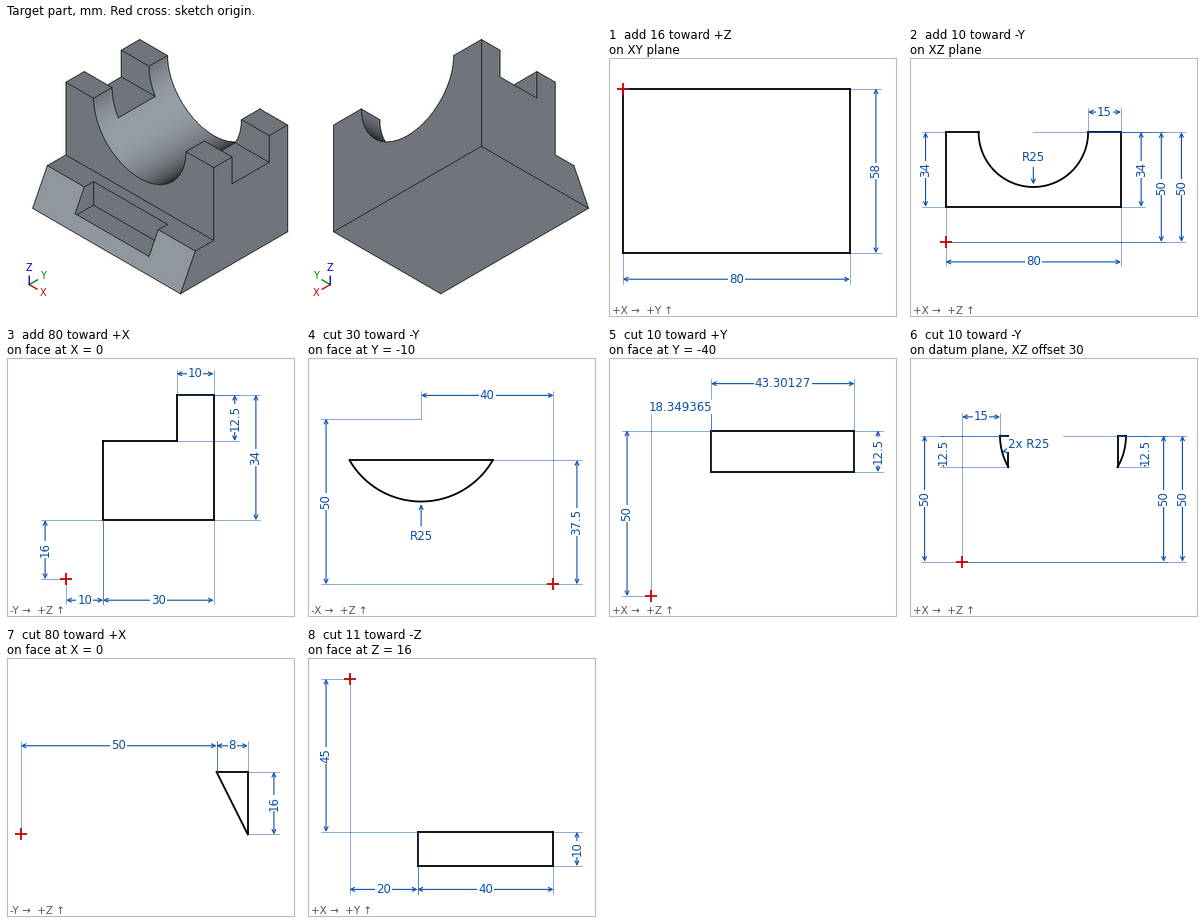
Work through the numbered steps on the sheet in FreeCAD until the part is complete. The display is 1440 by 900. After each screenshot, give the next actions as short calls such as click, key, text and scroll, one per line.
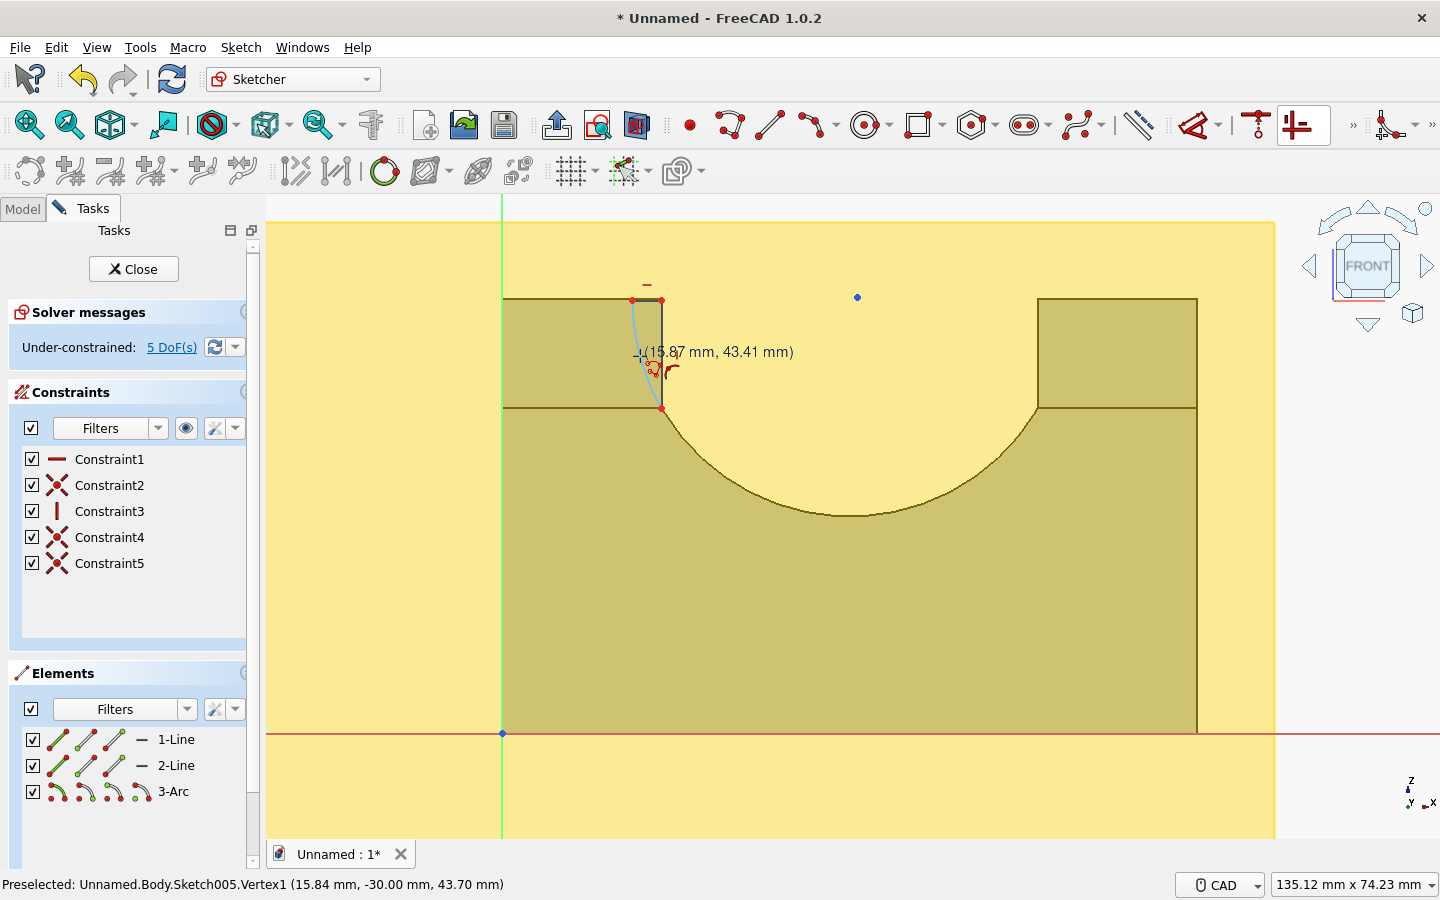
click(1038, 408)
click(1038, 299)
click(1067, 299)
right_click(1067, 299)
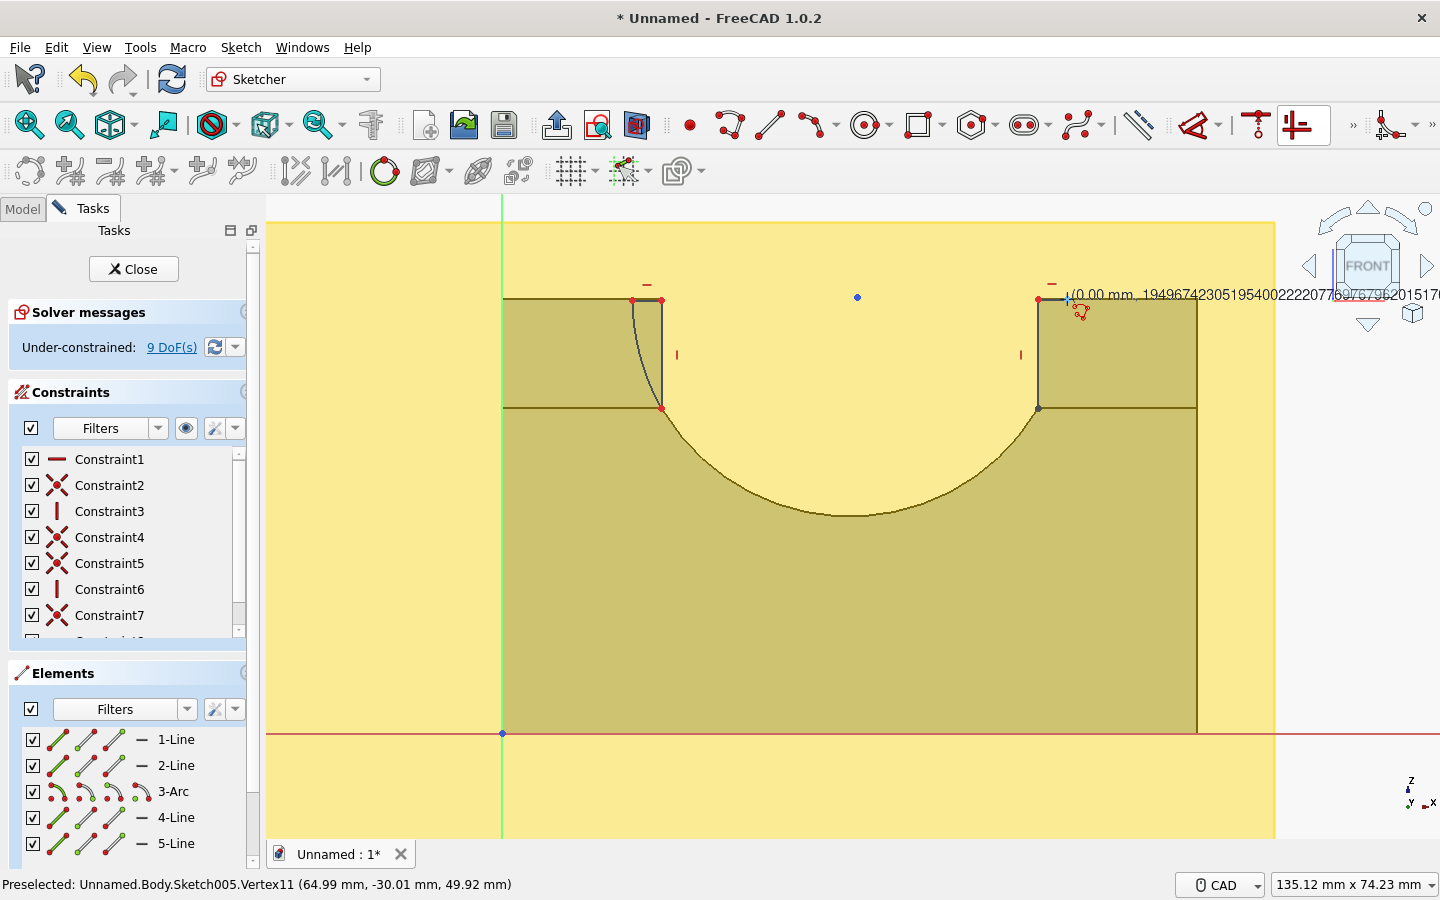
click(812, 126)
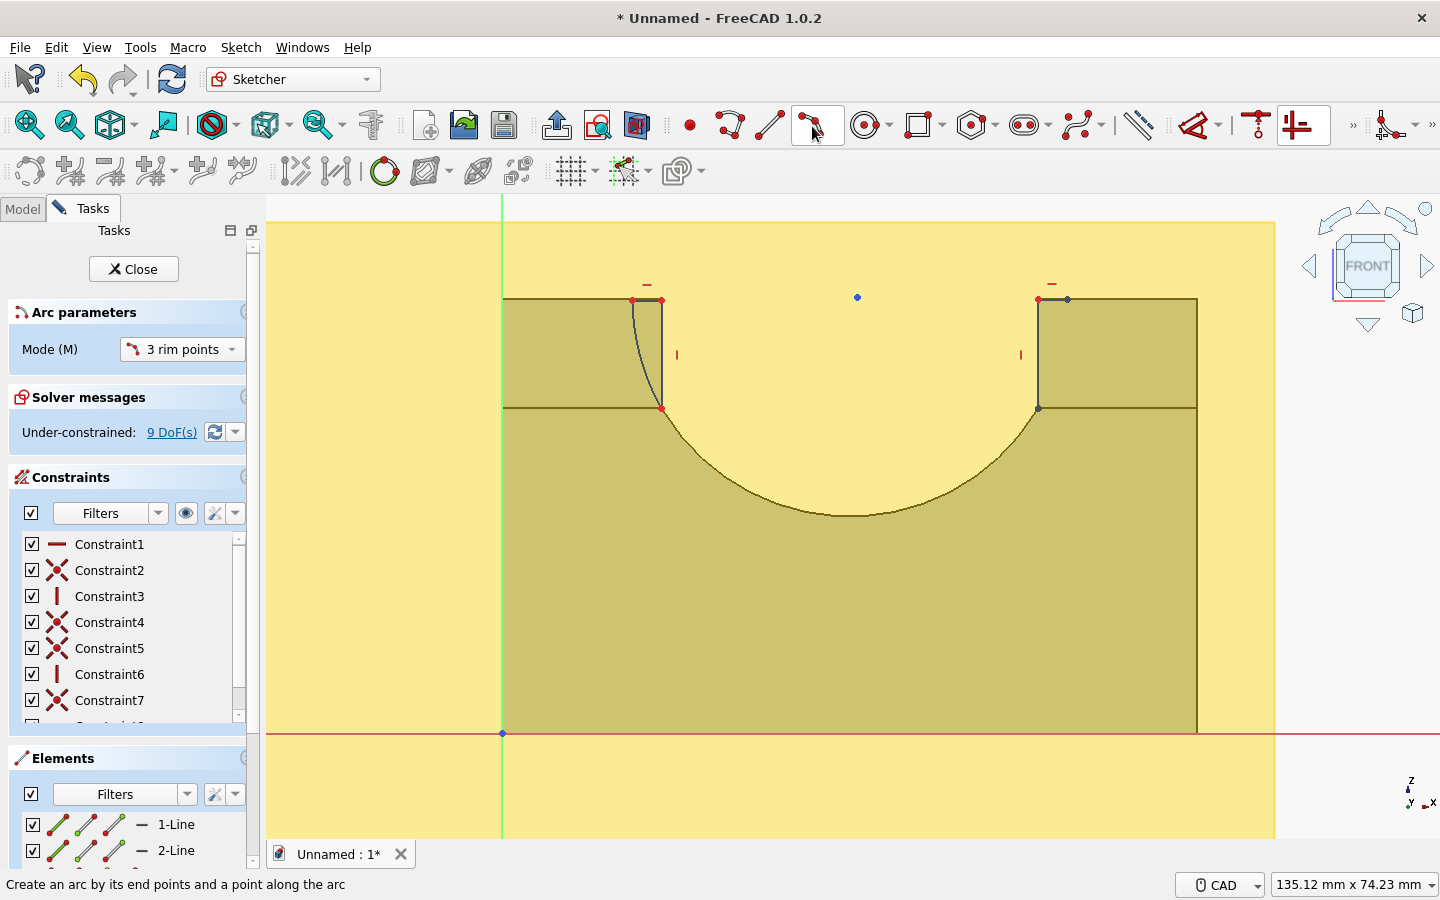
click(1067, 300)
click(1038, 409)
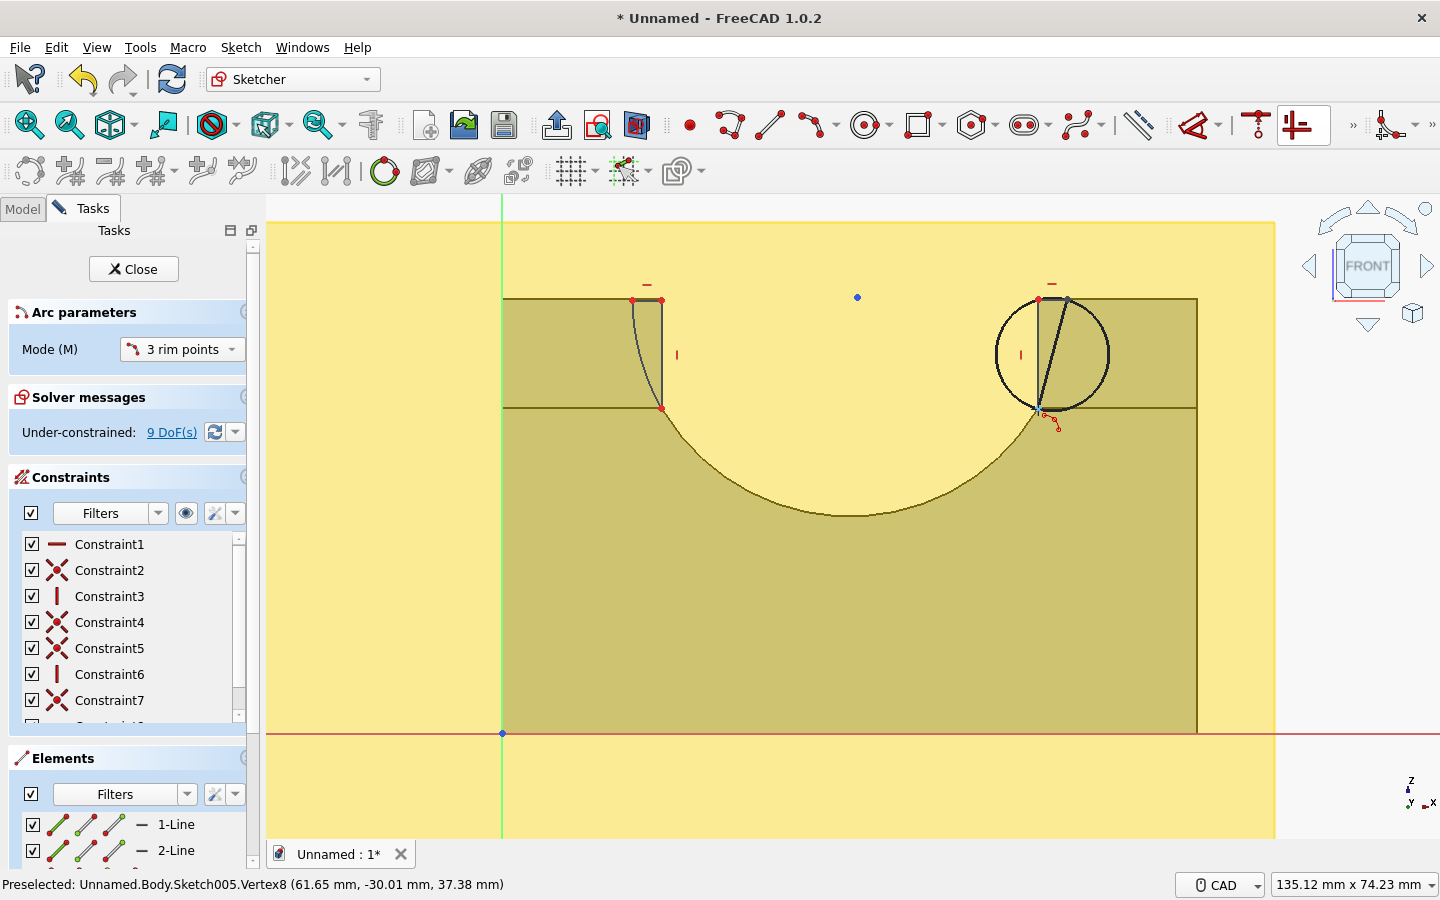
scroll(1060, 356, up, 4)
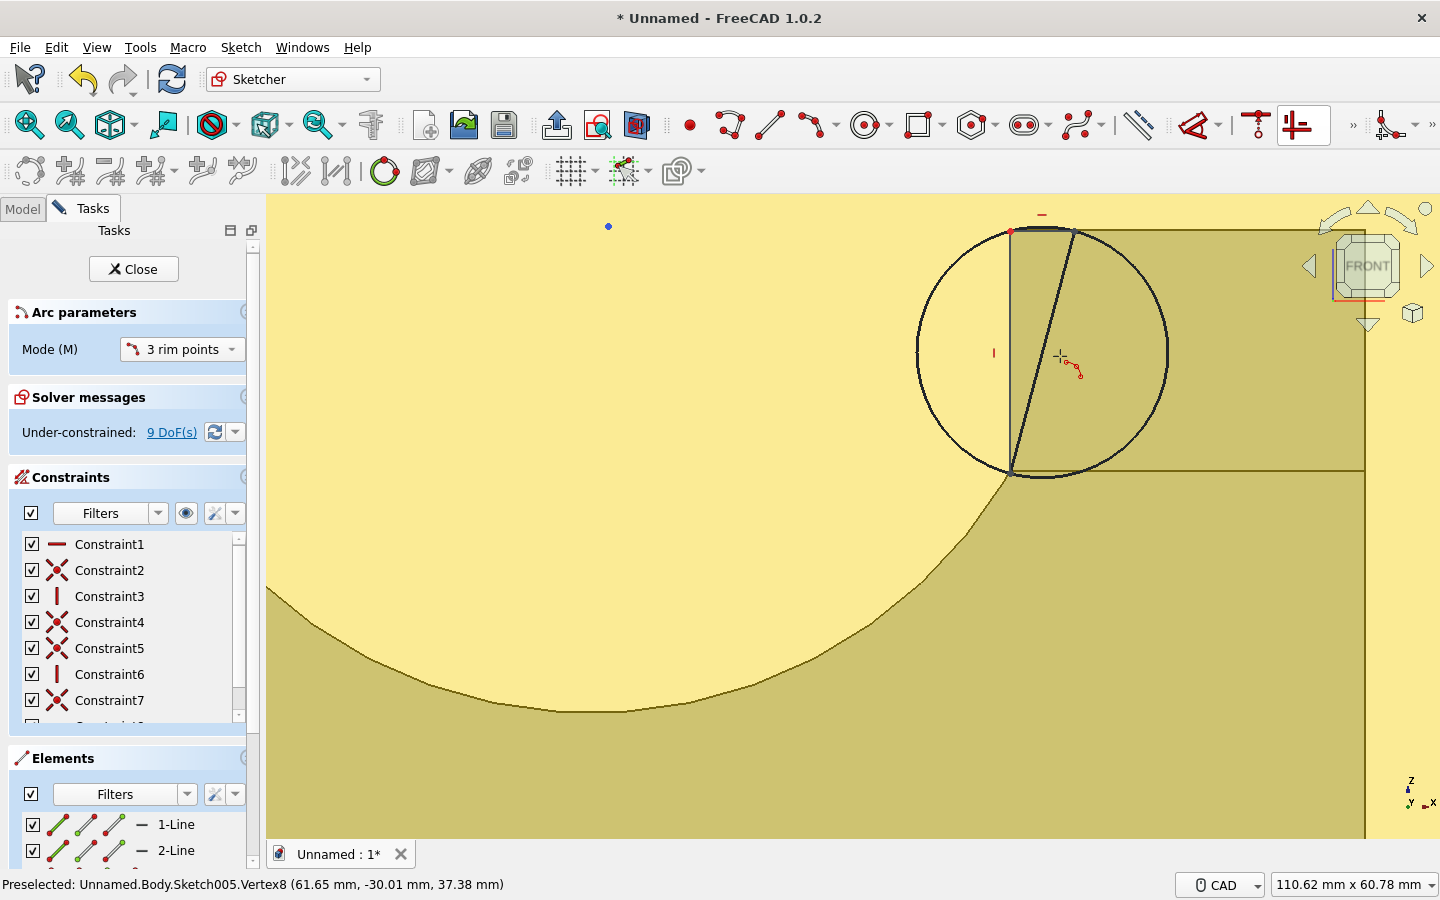
click(1058, 355)
key(Escape)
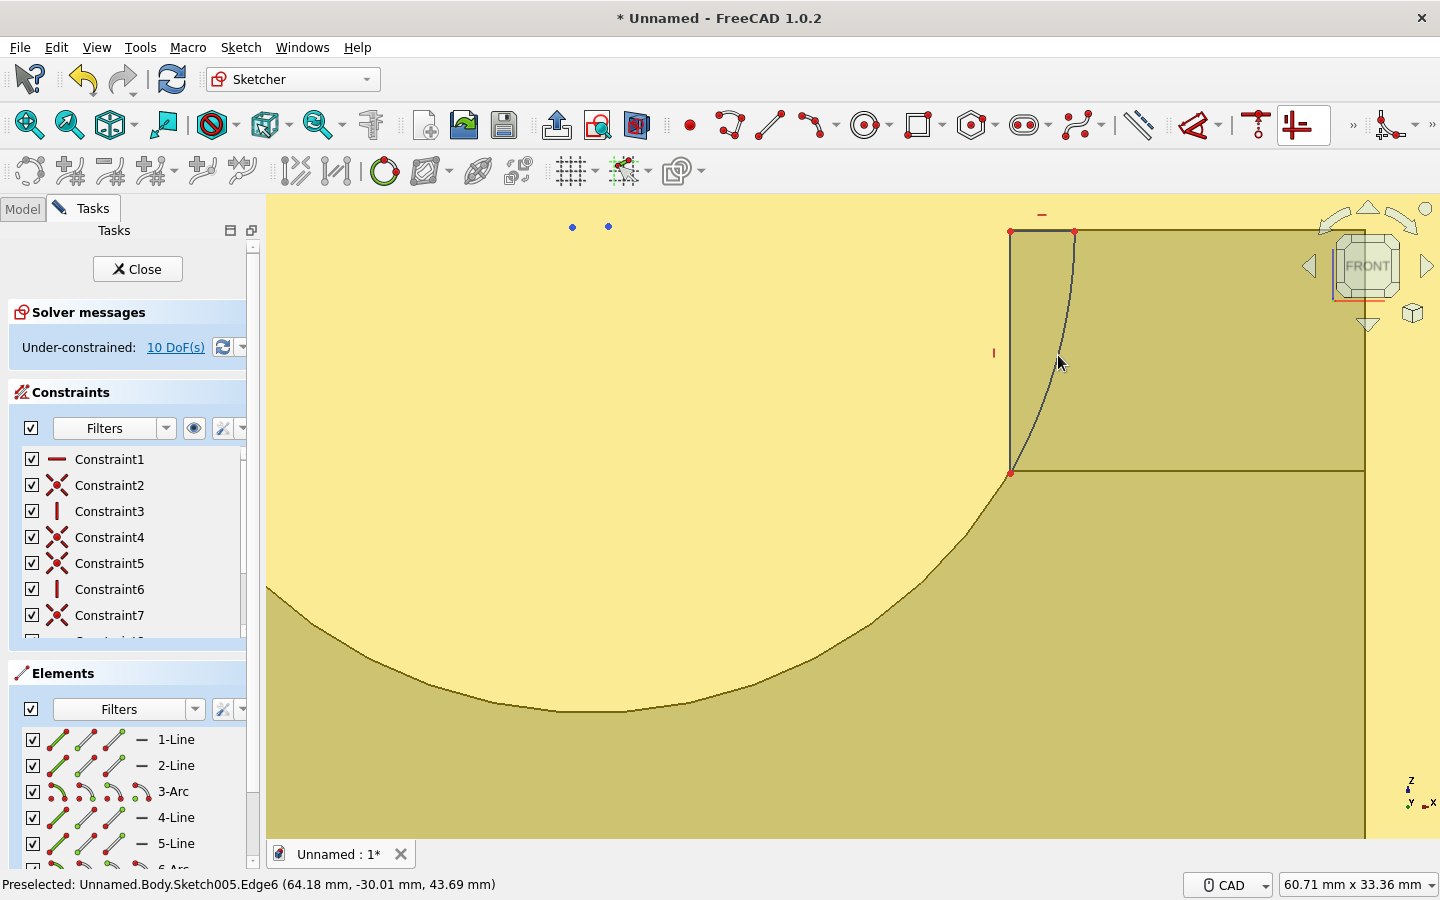
scroll(1060, 356, down, 4)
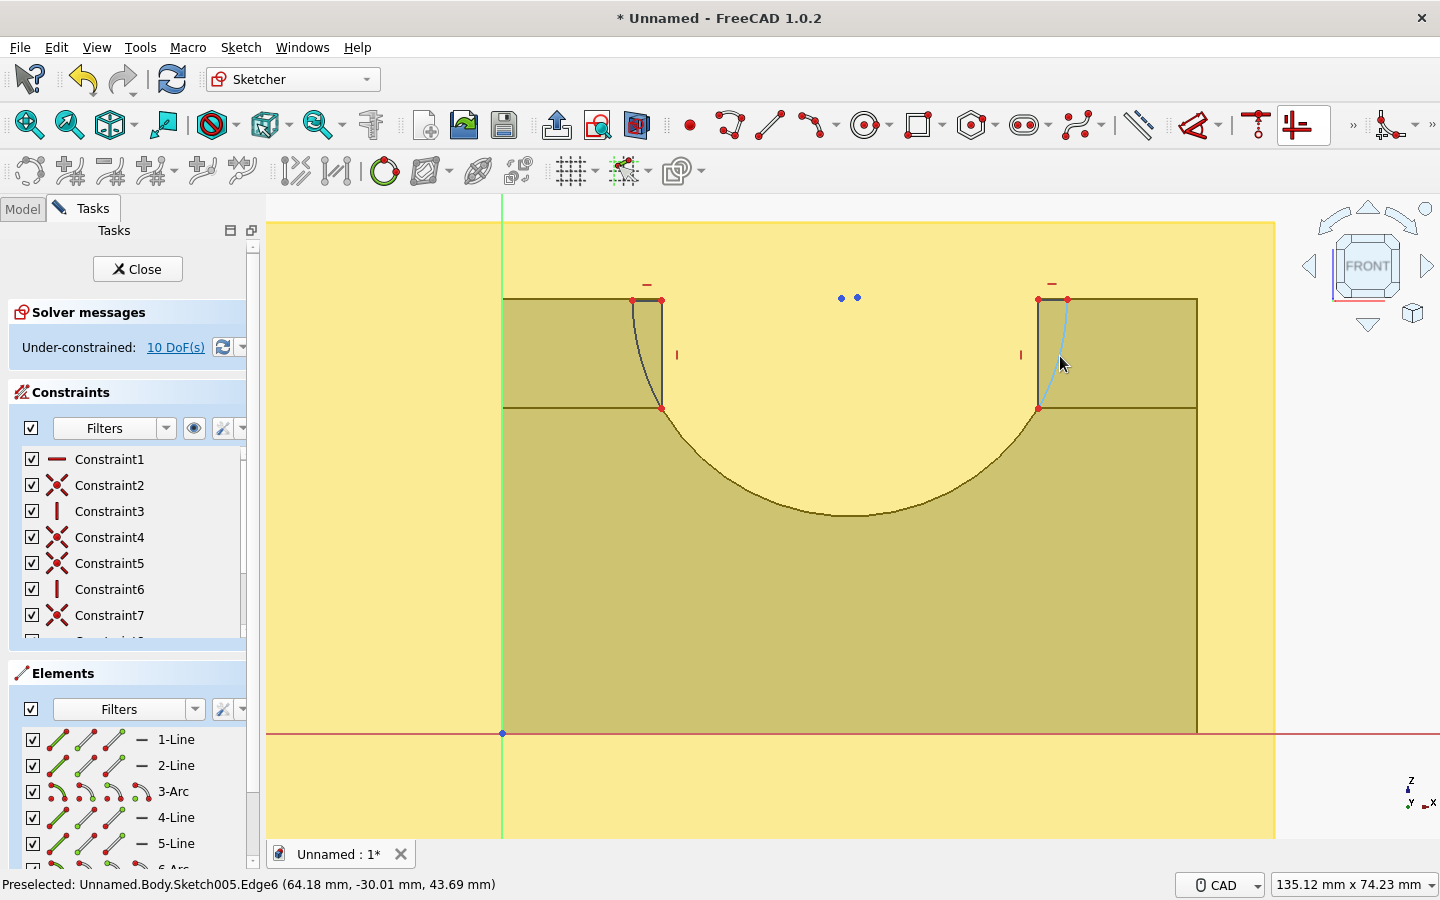
click(635, 334)